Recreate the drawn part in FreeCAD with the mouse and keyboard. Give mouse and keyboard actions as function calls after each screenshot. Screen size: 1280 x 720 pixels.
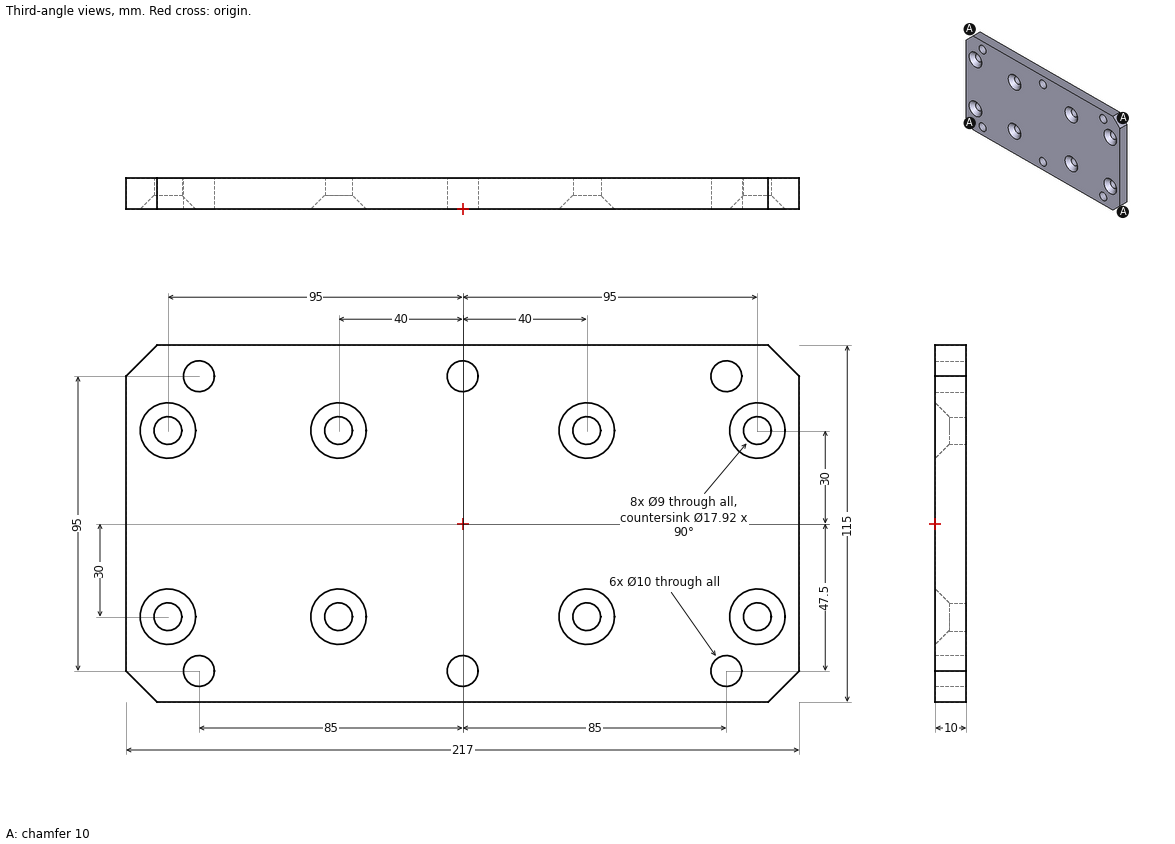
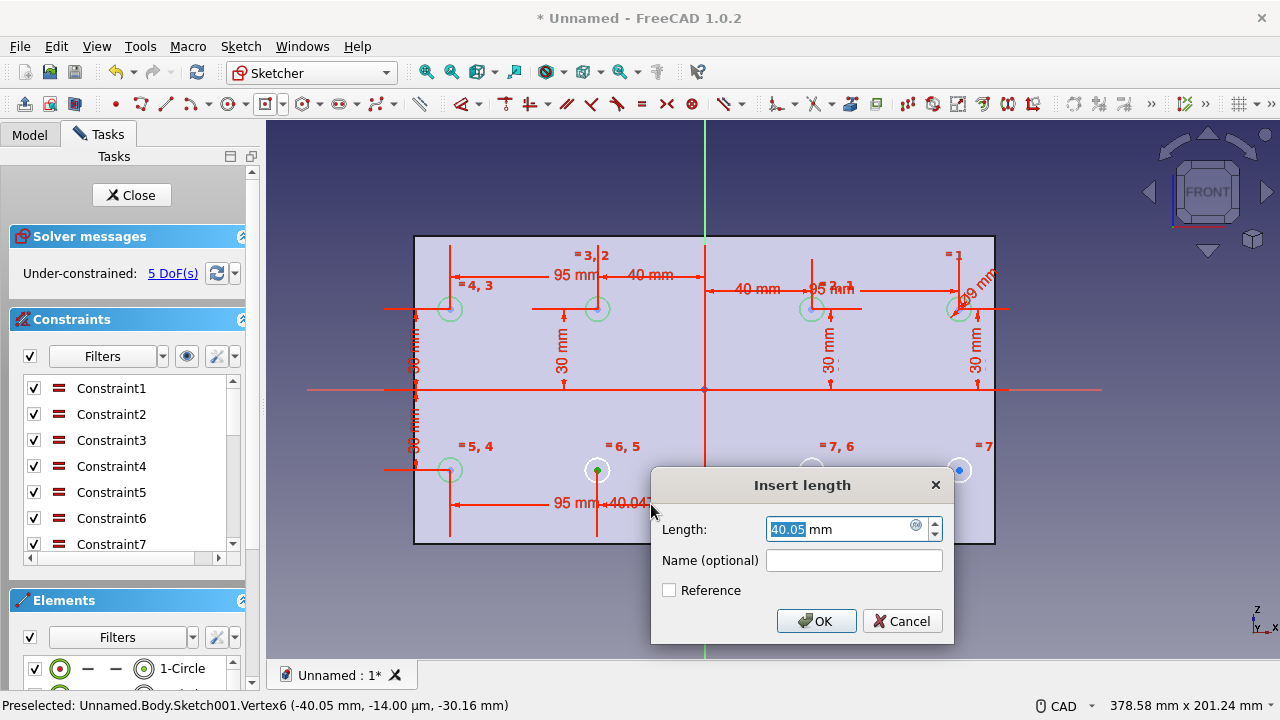
text(40)
key(Return)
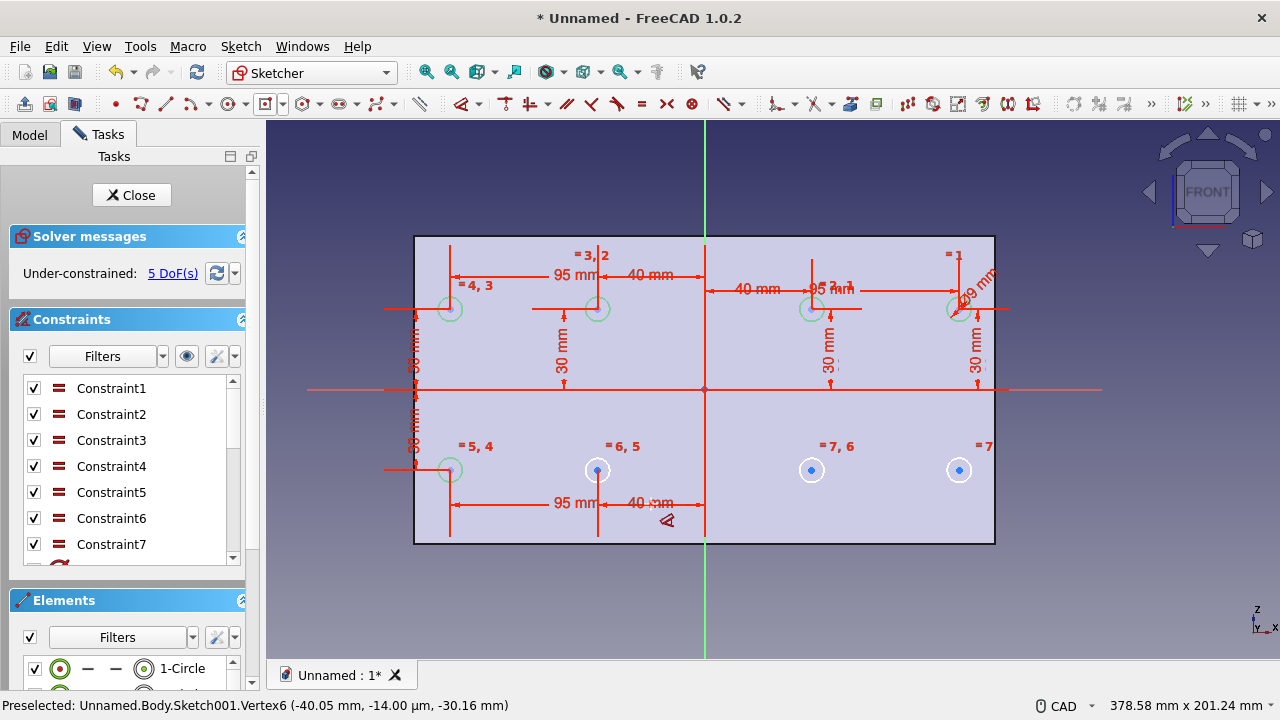
click(598, 470)
click(564, 430)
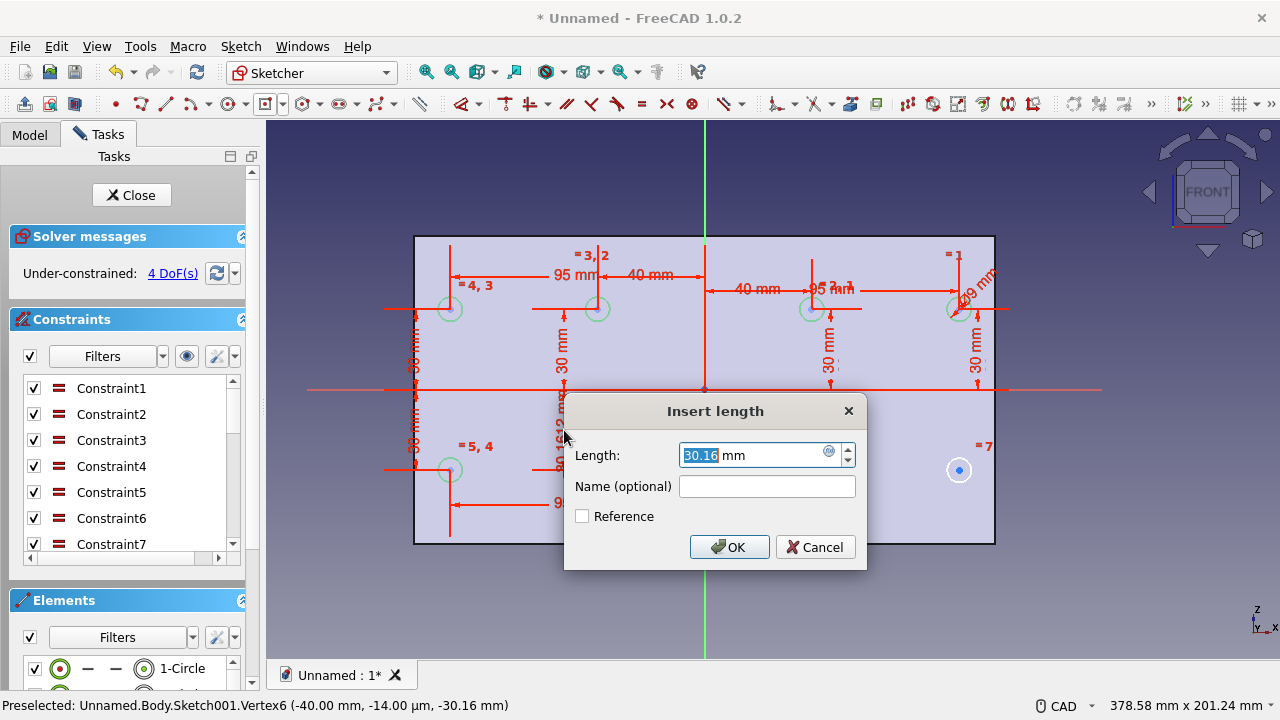
text(30)
key(Return)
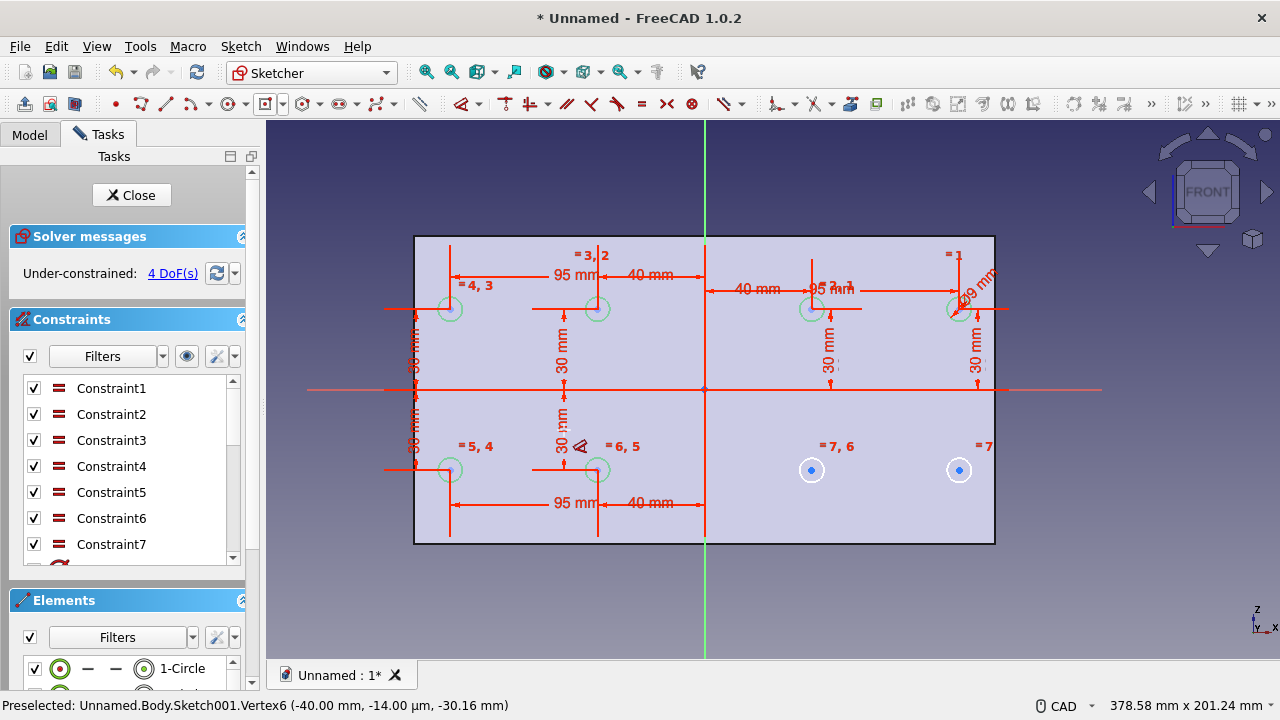
click(812, 470)
click(758, 504)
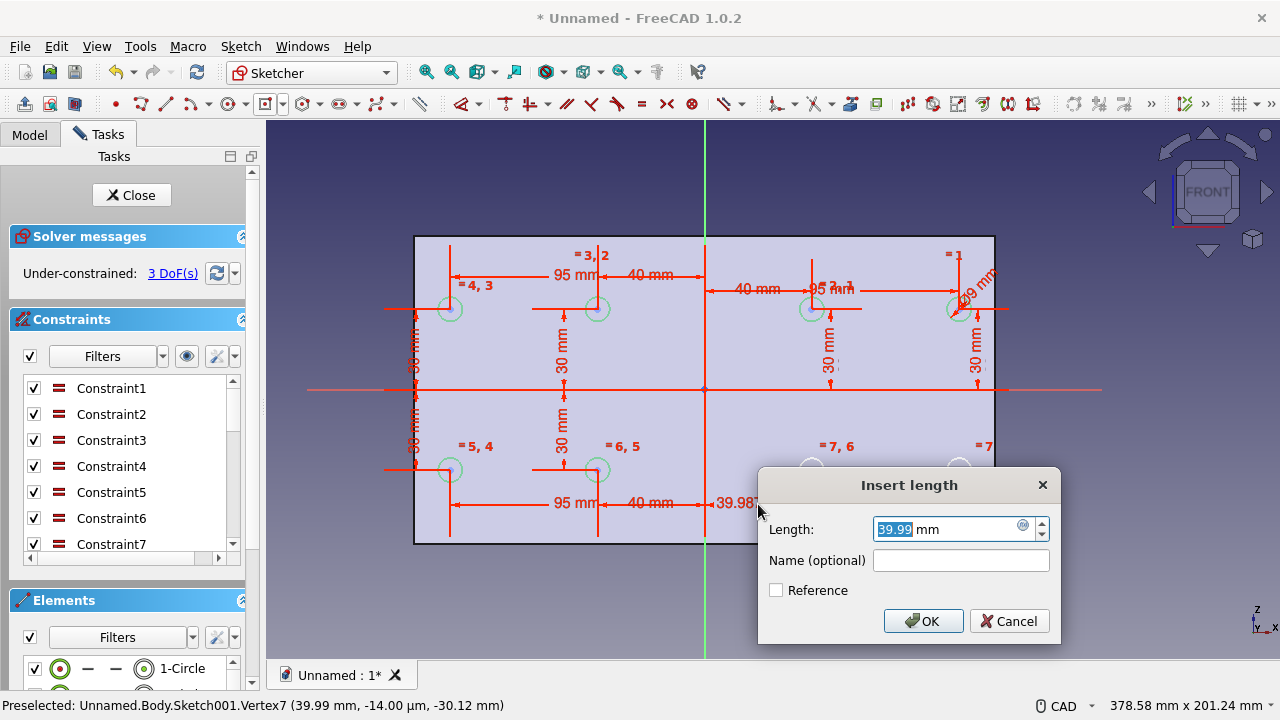
text(40)
key(Return)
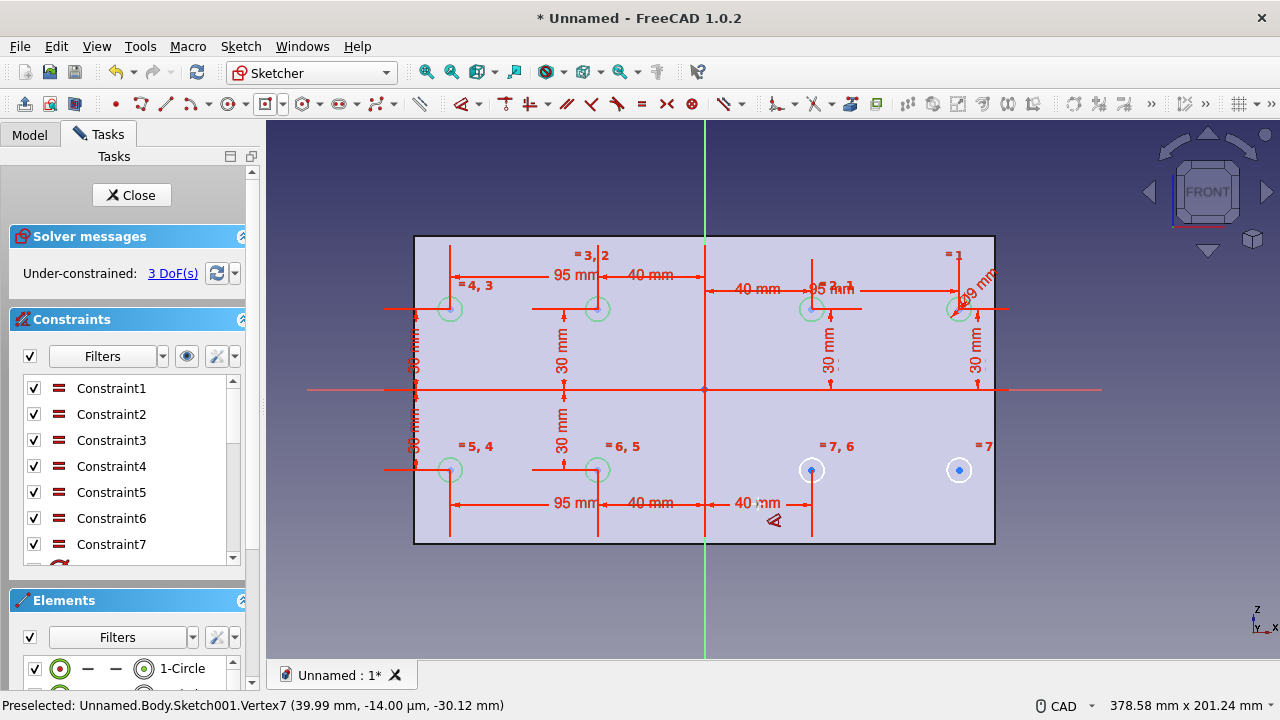
click(812, 470)
click(846, 430)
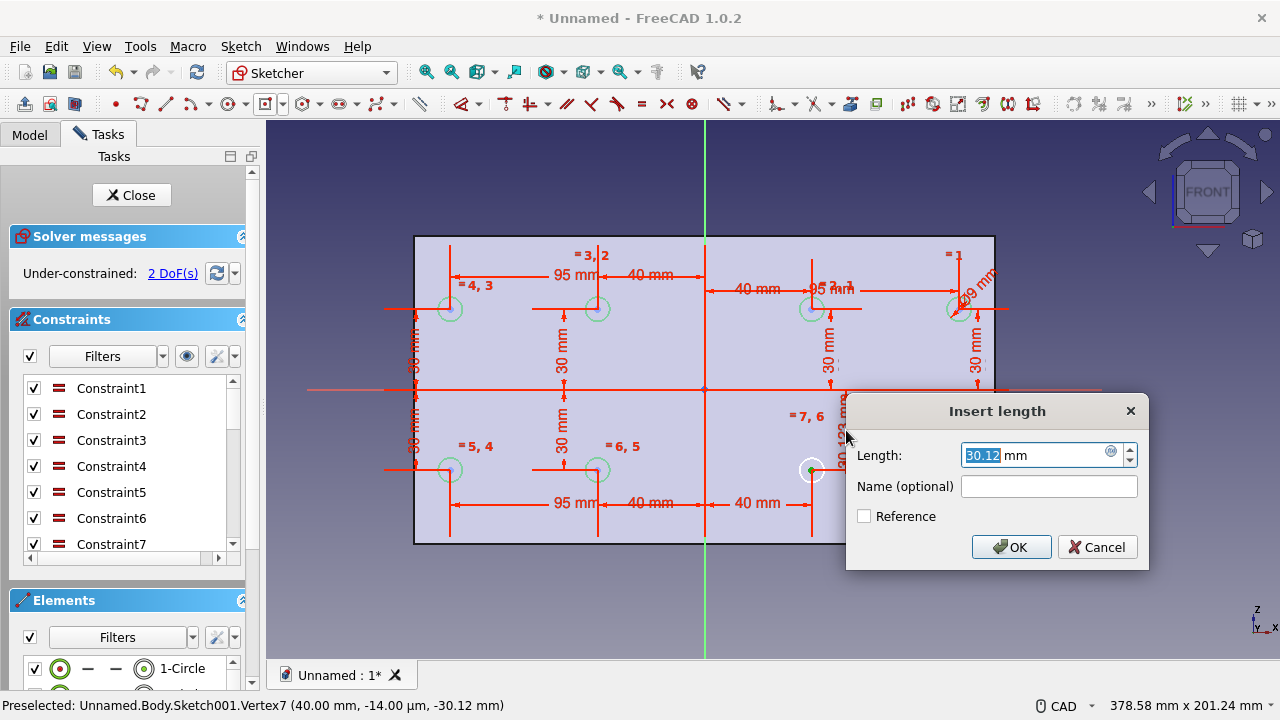
text(30)
key(Return)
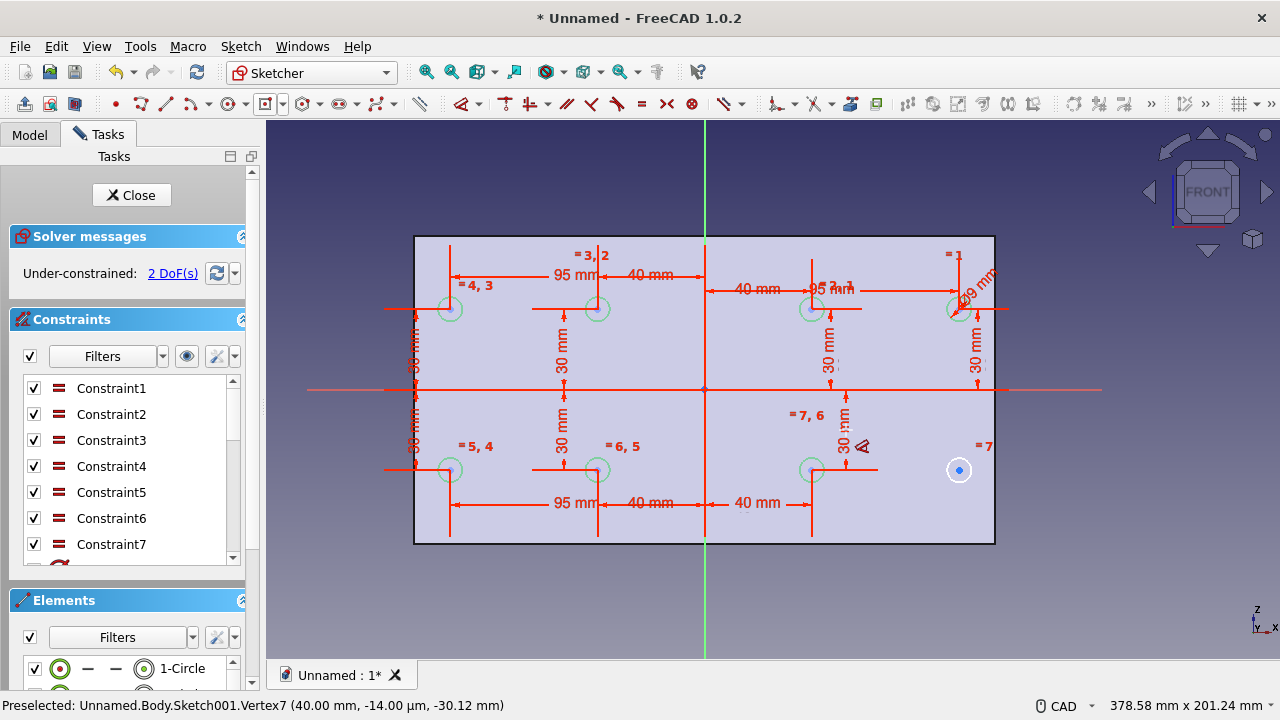
click(959, 470)
click(832, 504)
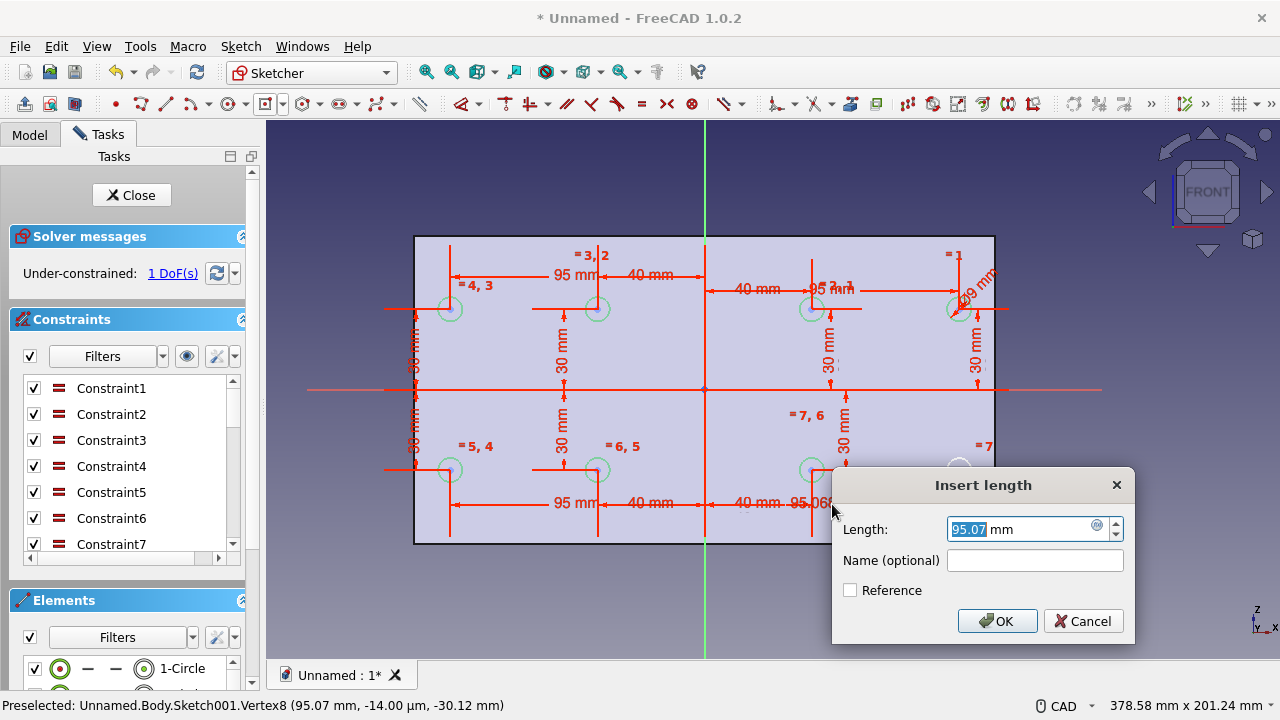
text(95)
key(Return)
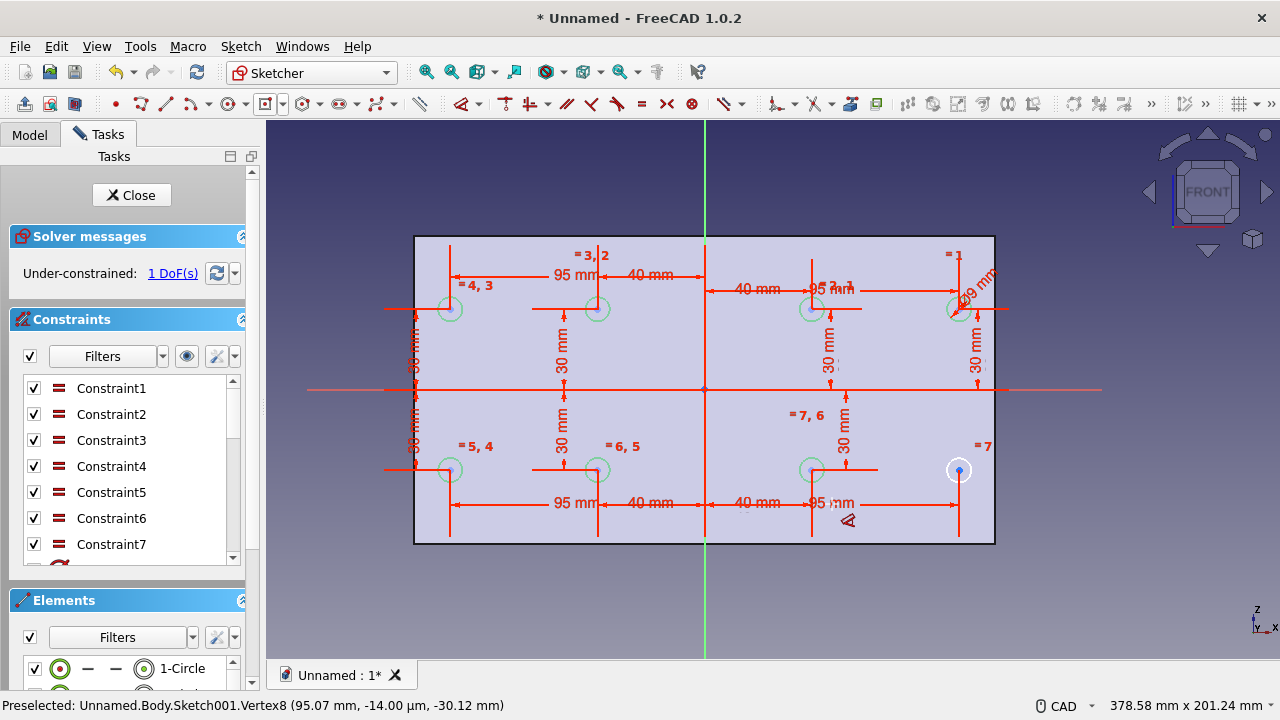
click(959, 470)
click(993, 430)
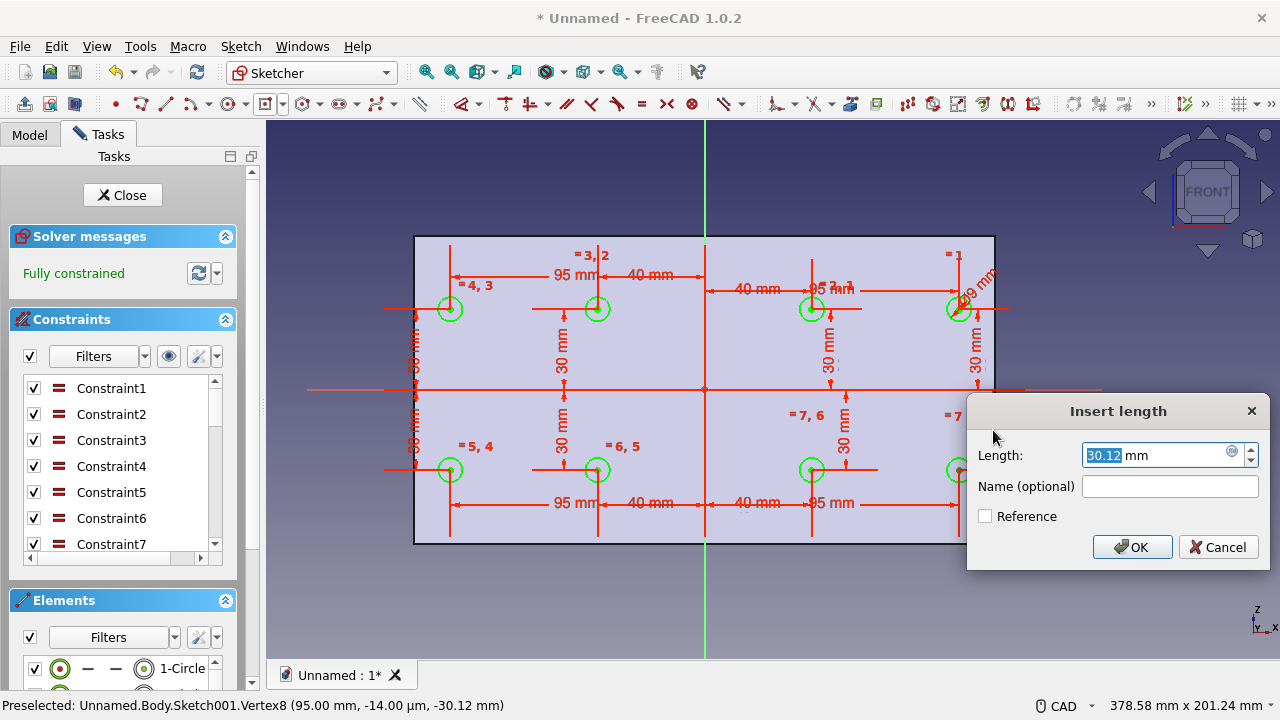
text(30)
key(Return)
key(Escape)